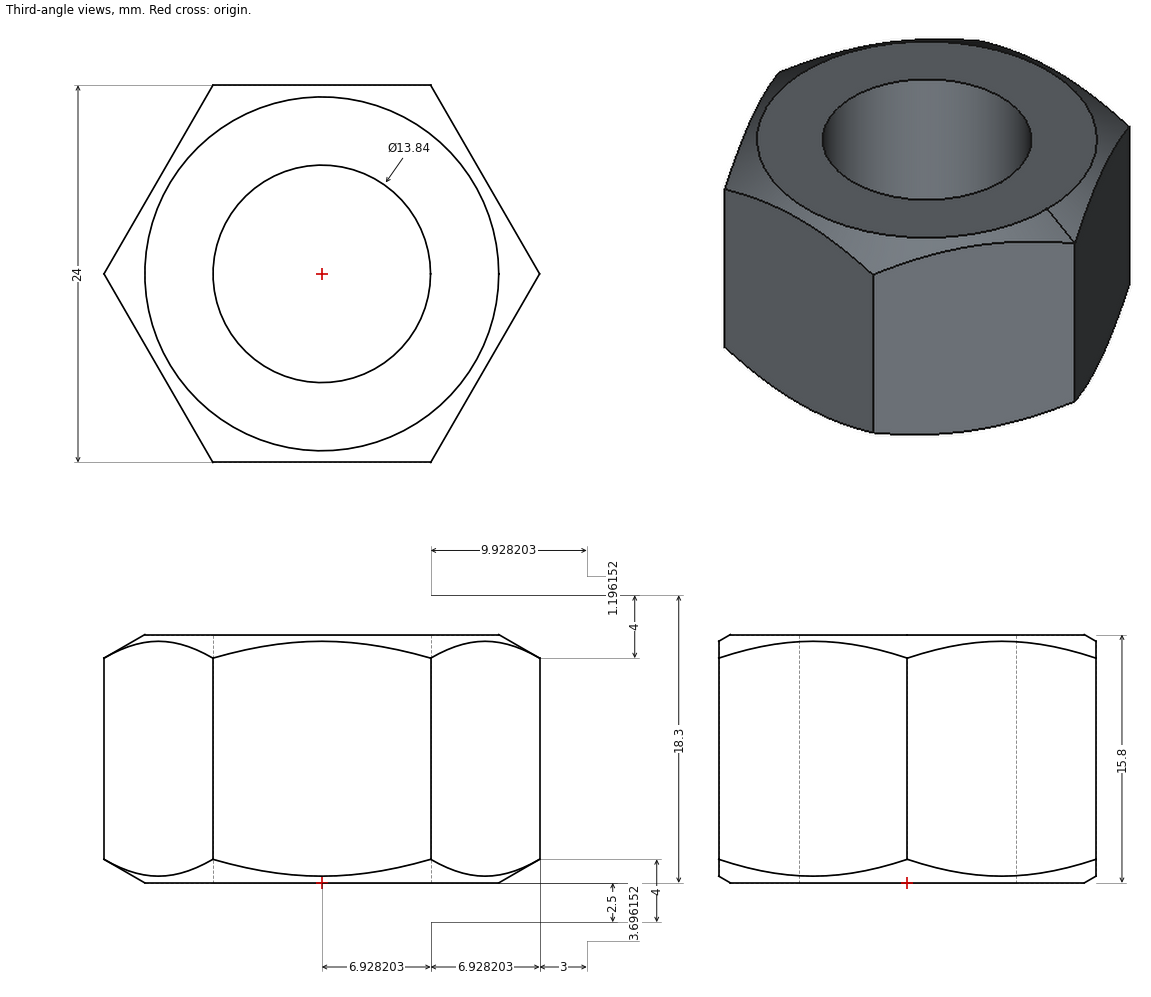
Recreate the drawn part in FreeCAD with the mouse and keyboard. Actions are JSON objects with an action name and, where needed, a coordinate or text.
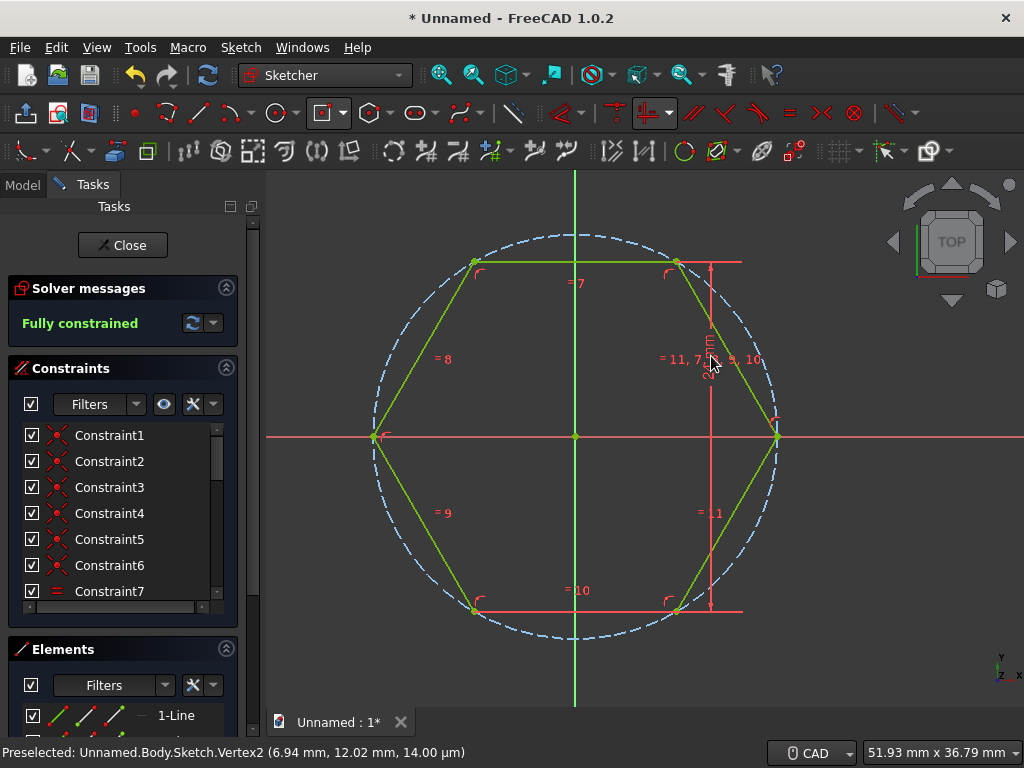
{"action": "left_click", "coordinate": [123, 245]}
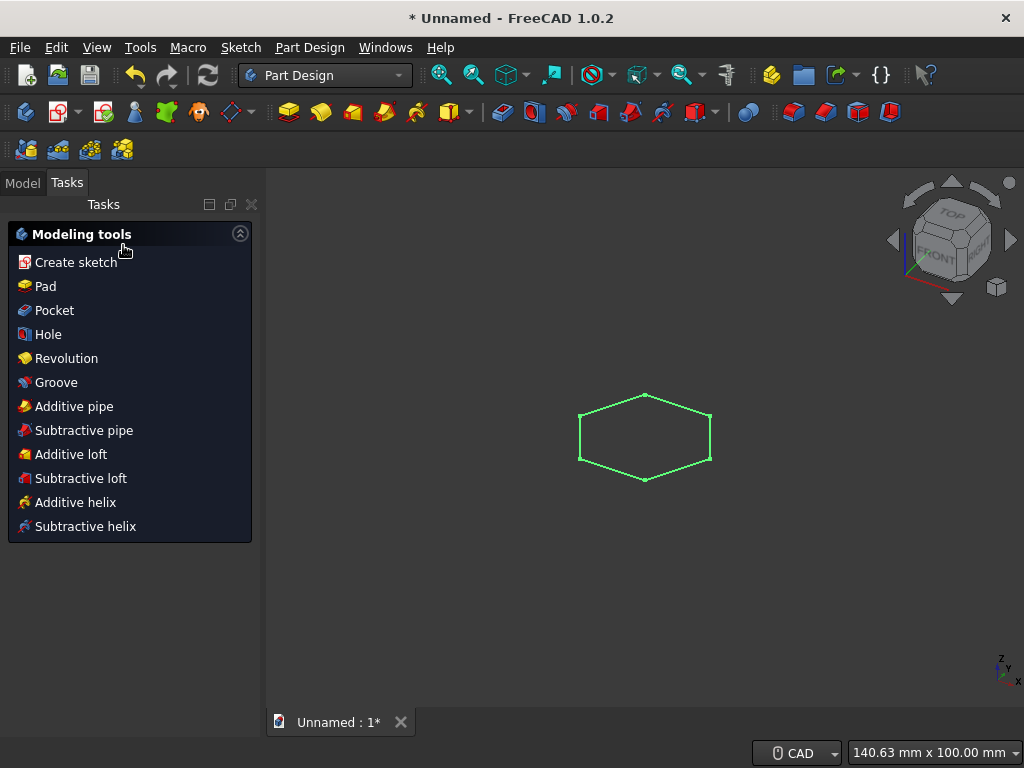
{"action": "left_click", "coordinate": [290, 112]}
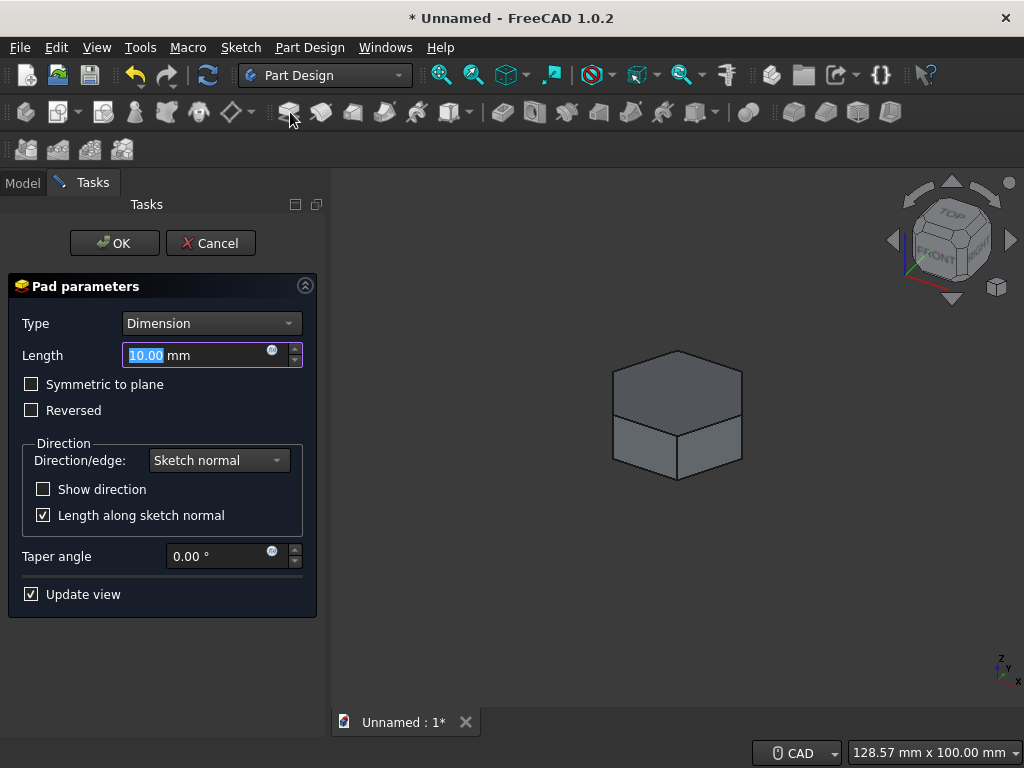
{"action": "type", "text": "15.8"}
{"action": "key", "text": "Tab"}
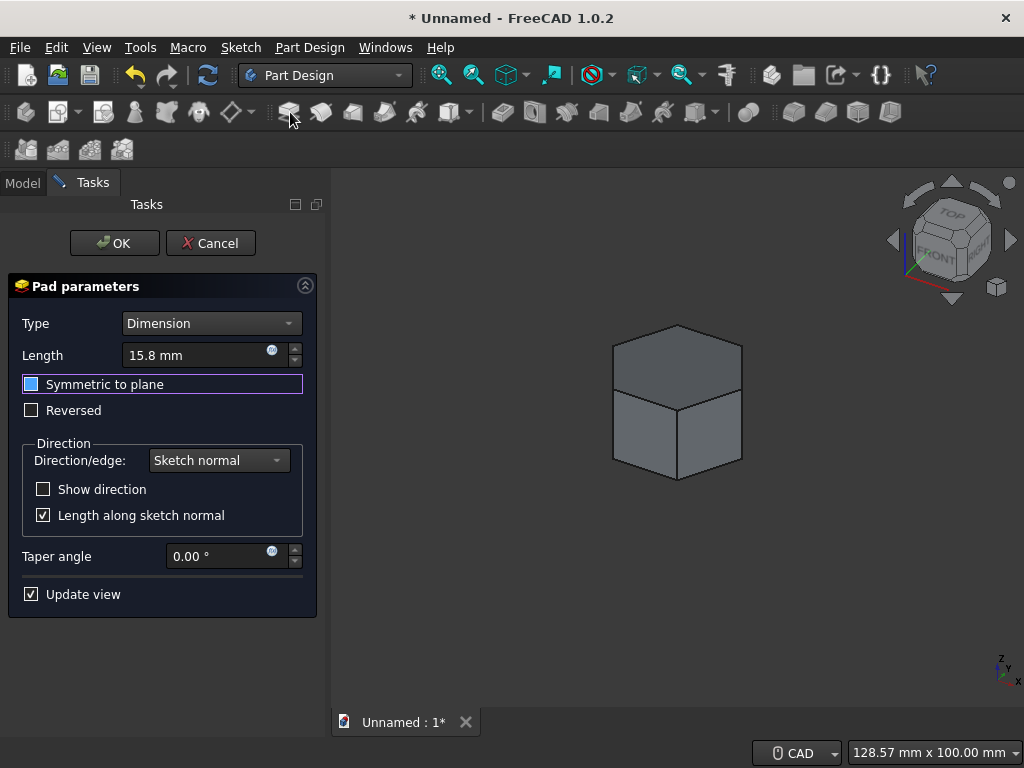
{"action": "left_click", "coordinate": [115, 243]}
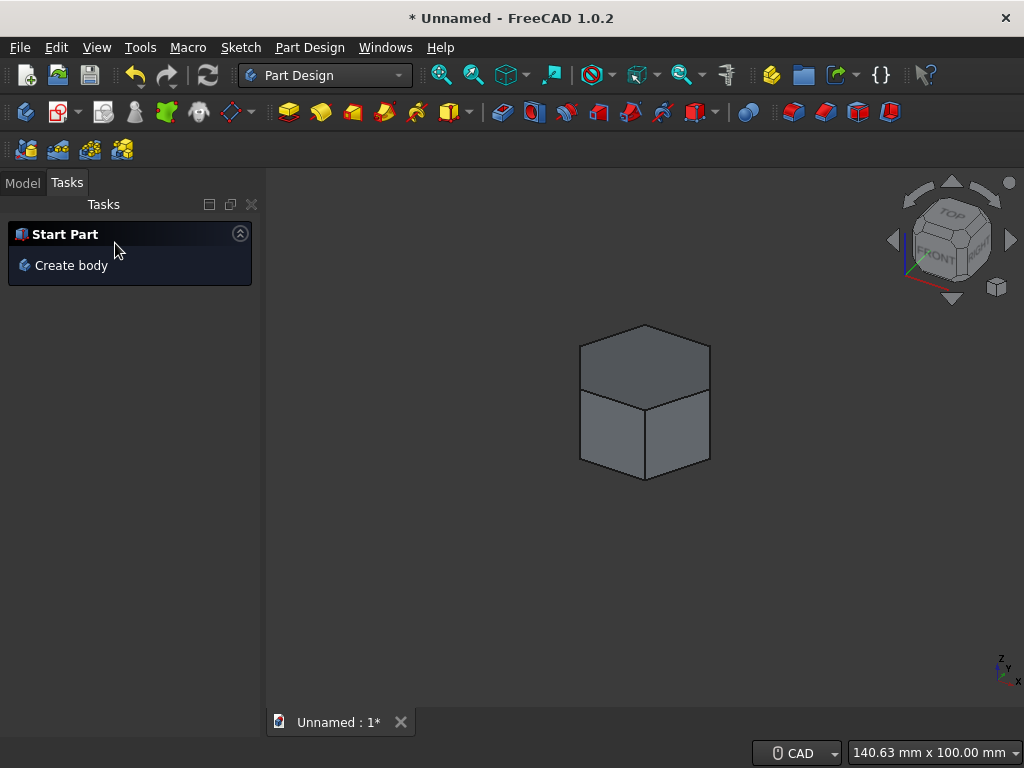
{"action": "left_click", "coordinate": [442, 76]}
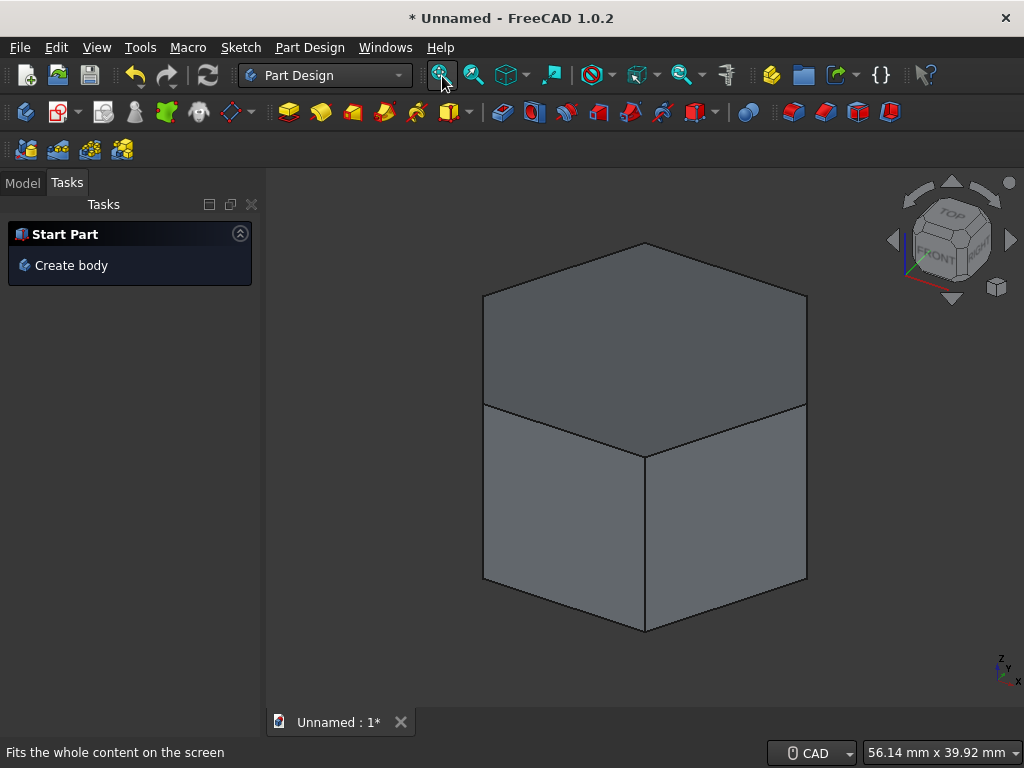
{"action": "left_click", "coordinate": [58, 112]}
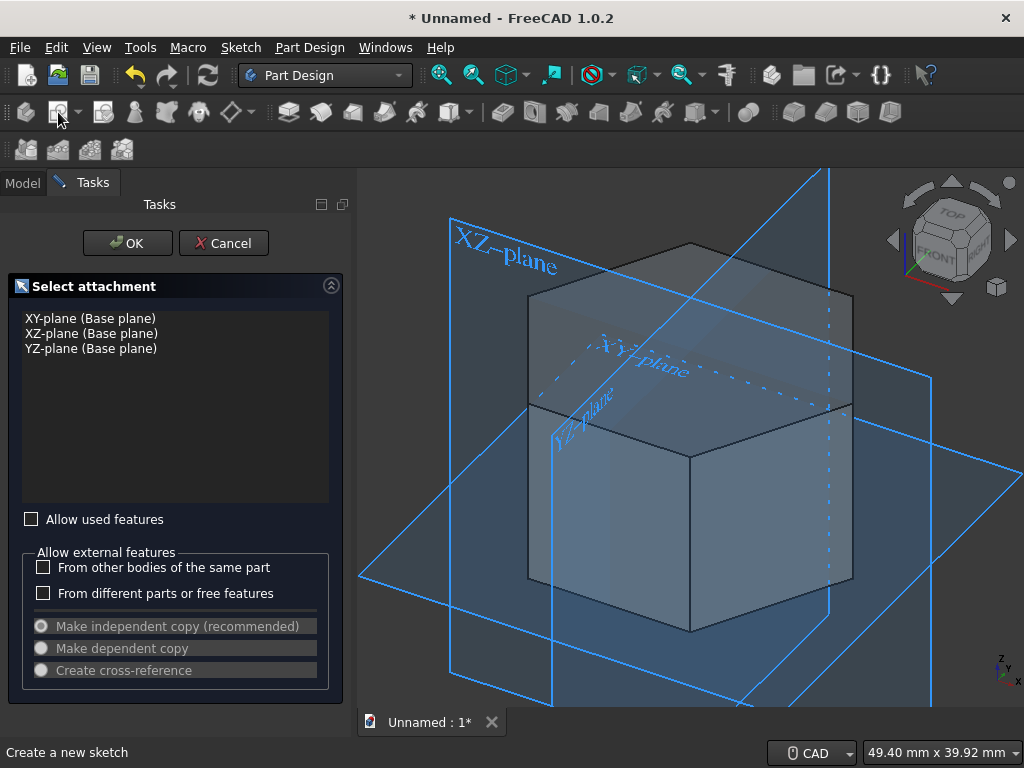
{"action": "left_click", "coordinate": [82, 334]}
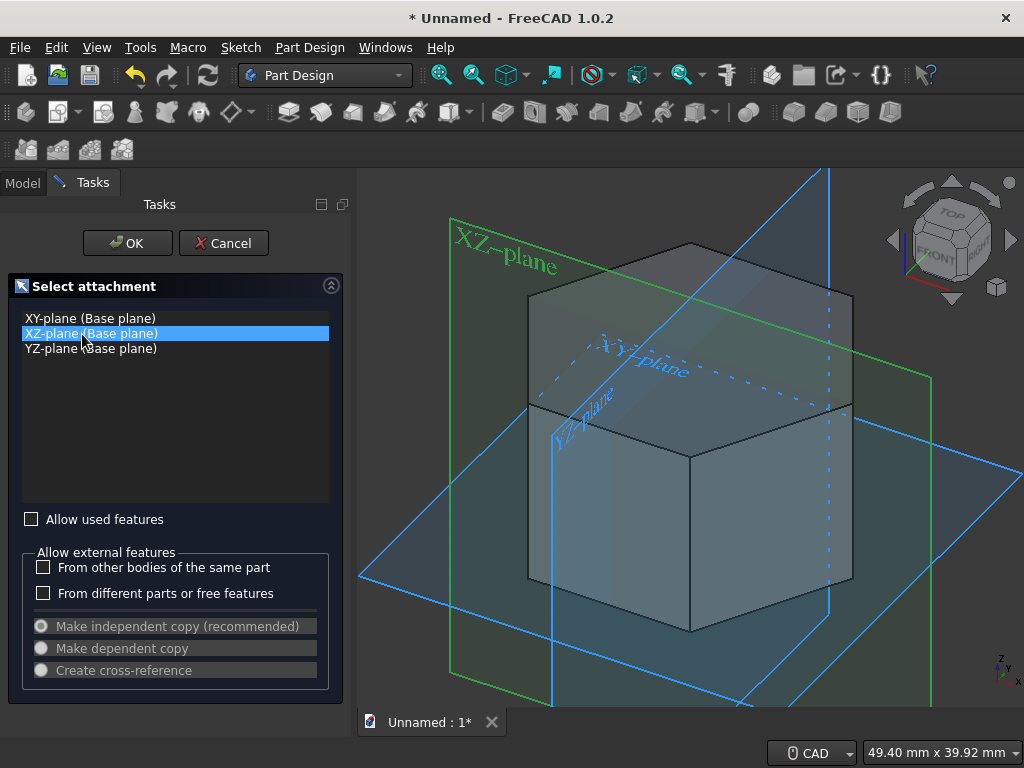
{"action": "left_click", "coordinate": [128, 243]}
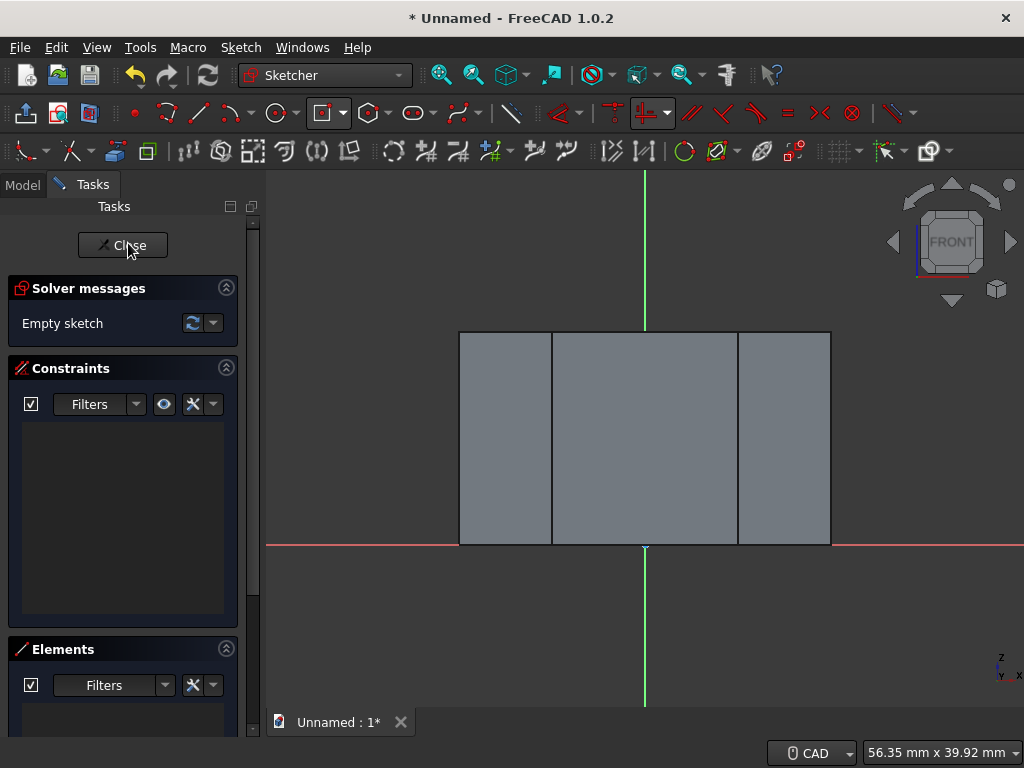
{"action": "left_click", "coordinate": [90, 114]}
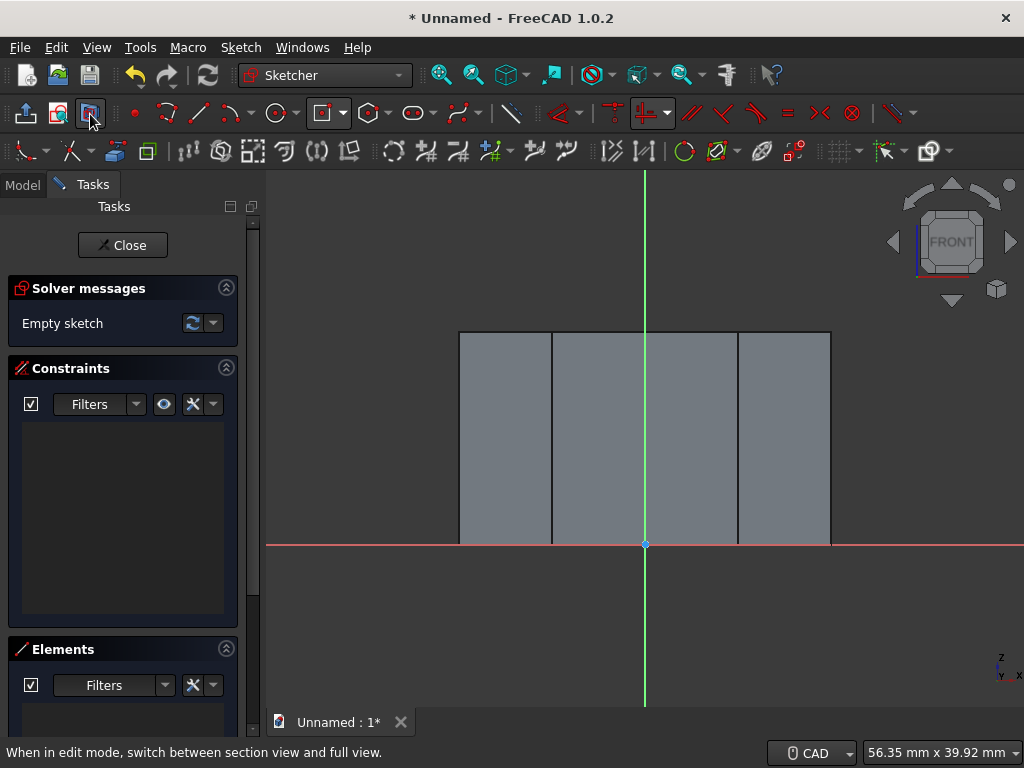
{"action": "scroll", "coordinate": [294, 439], "scroll_direction": "down", "scroll_amount": 1}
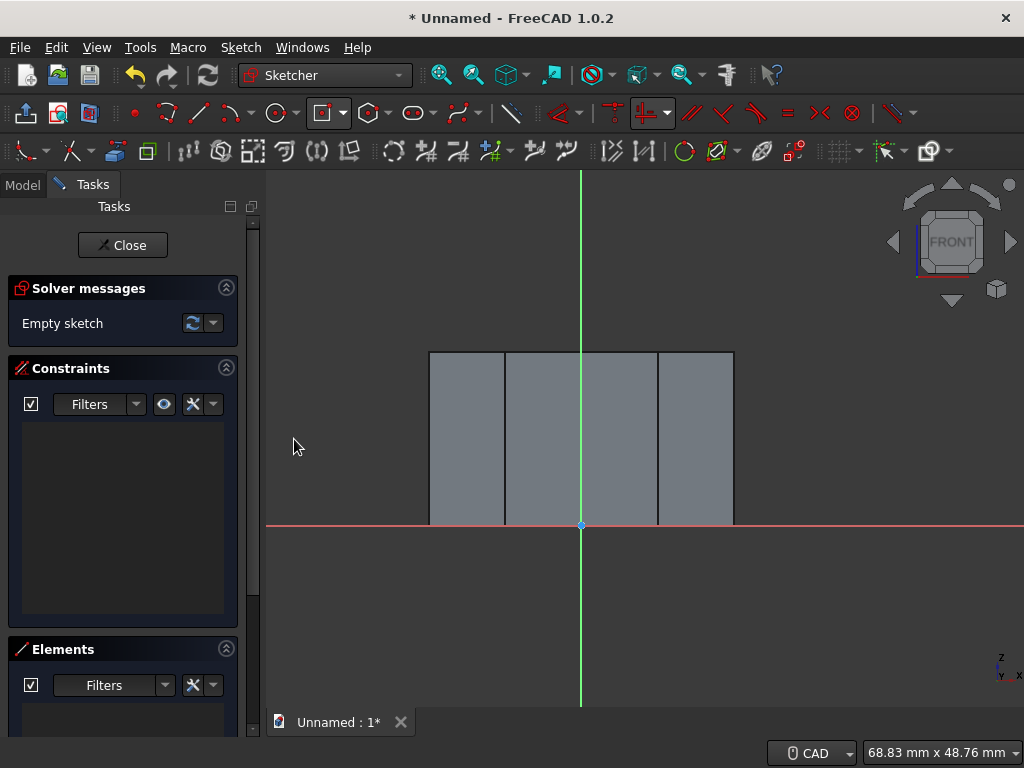
{"action": "left_click", "coordinate": [168, 114]}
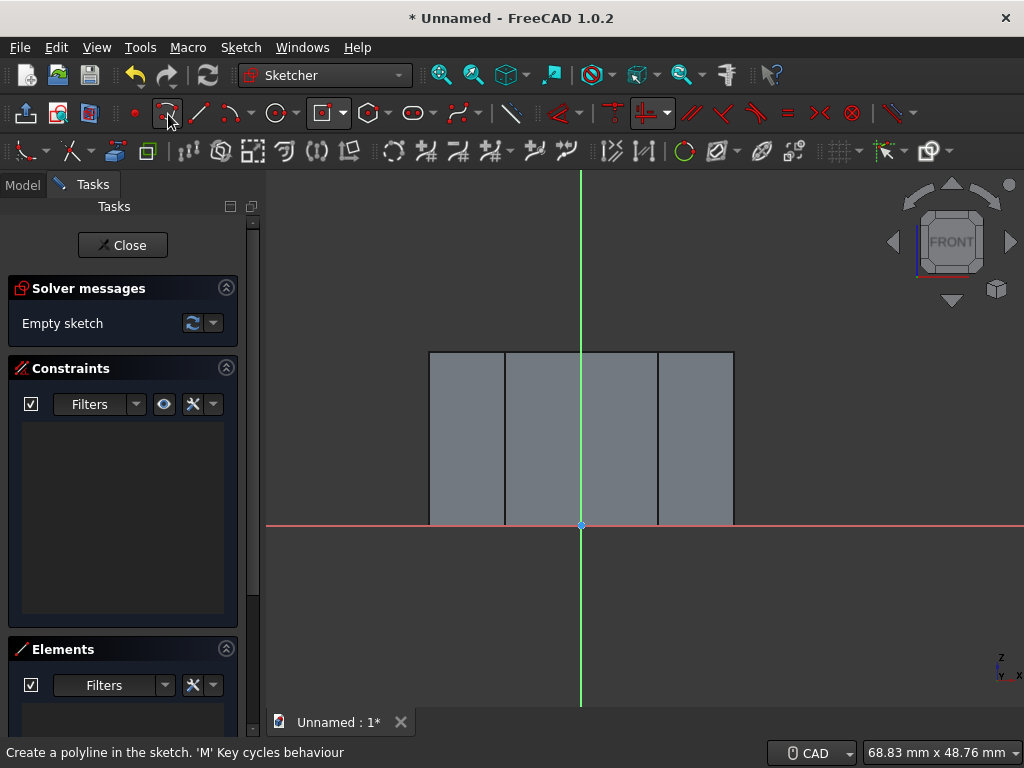
{"action": "left_click", "coordinate": [658, 553]}
{"action": "left_click", "coordinate": [734, 509]}
{"action": "left_click", "coordinate": [767, 566]}
{"action": "left_click", "coordinate": [658, 554]}